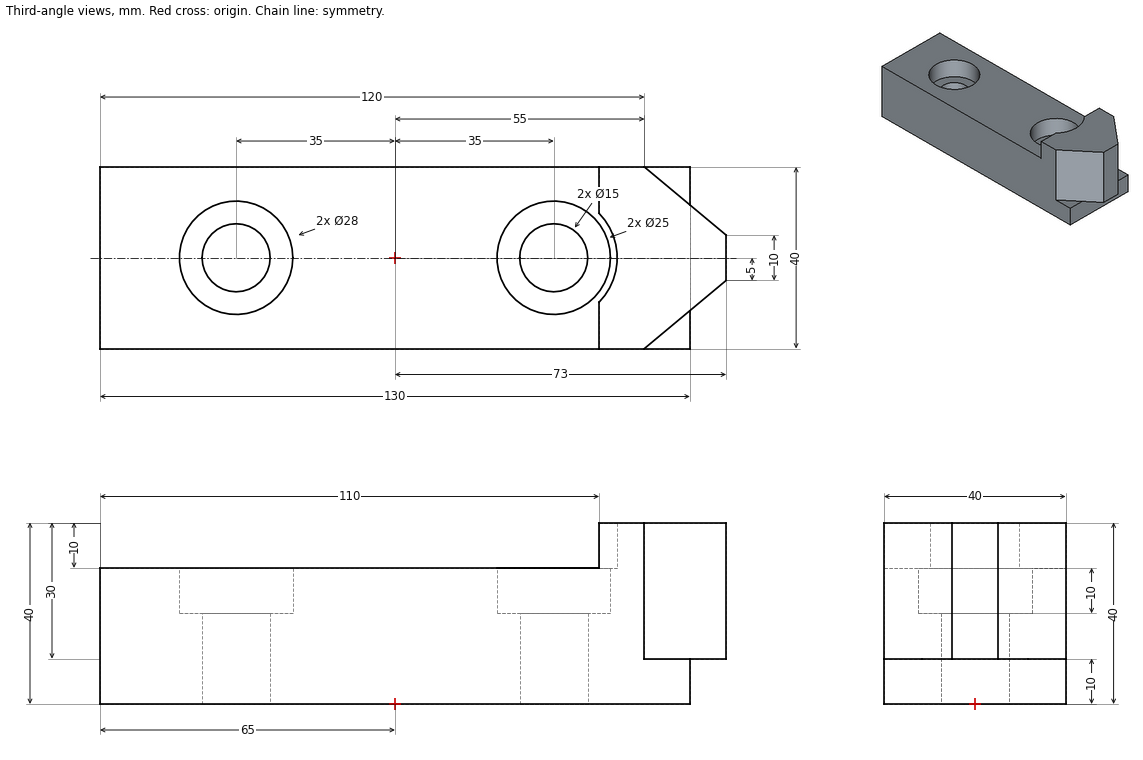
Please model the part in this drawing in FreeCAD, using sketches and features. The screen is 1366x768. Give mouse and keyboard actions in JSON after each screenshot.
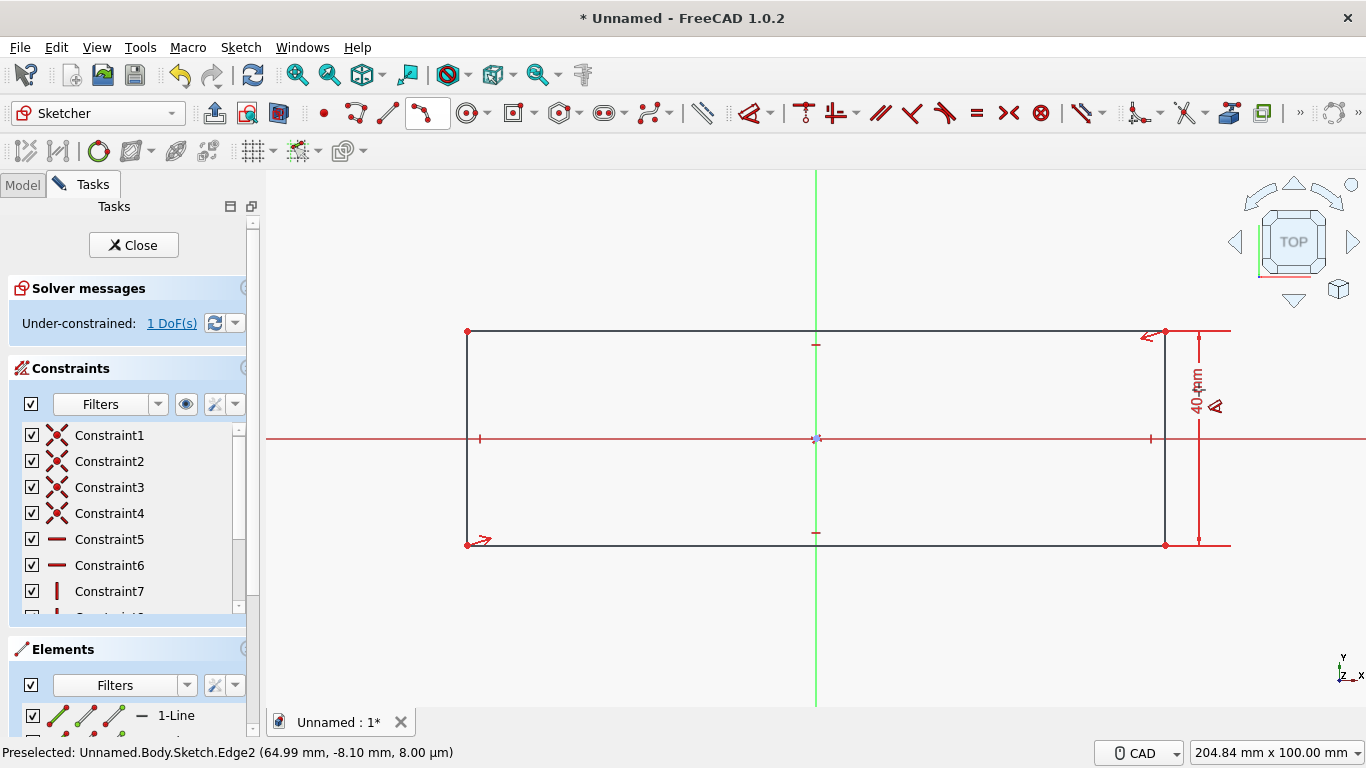
{"action": "left_click", "coordinate": [676, 546]}
{"action": "left_click", "coordinate": [655, 580]}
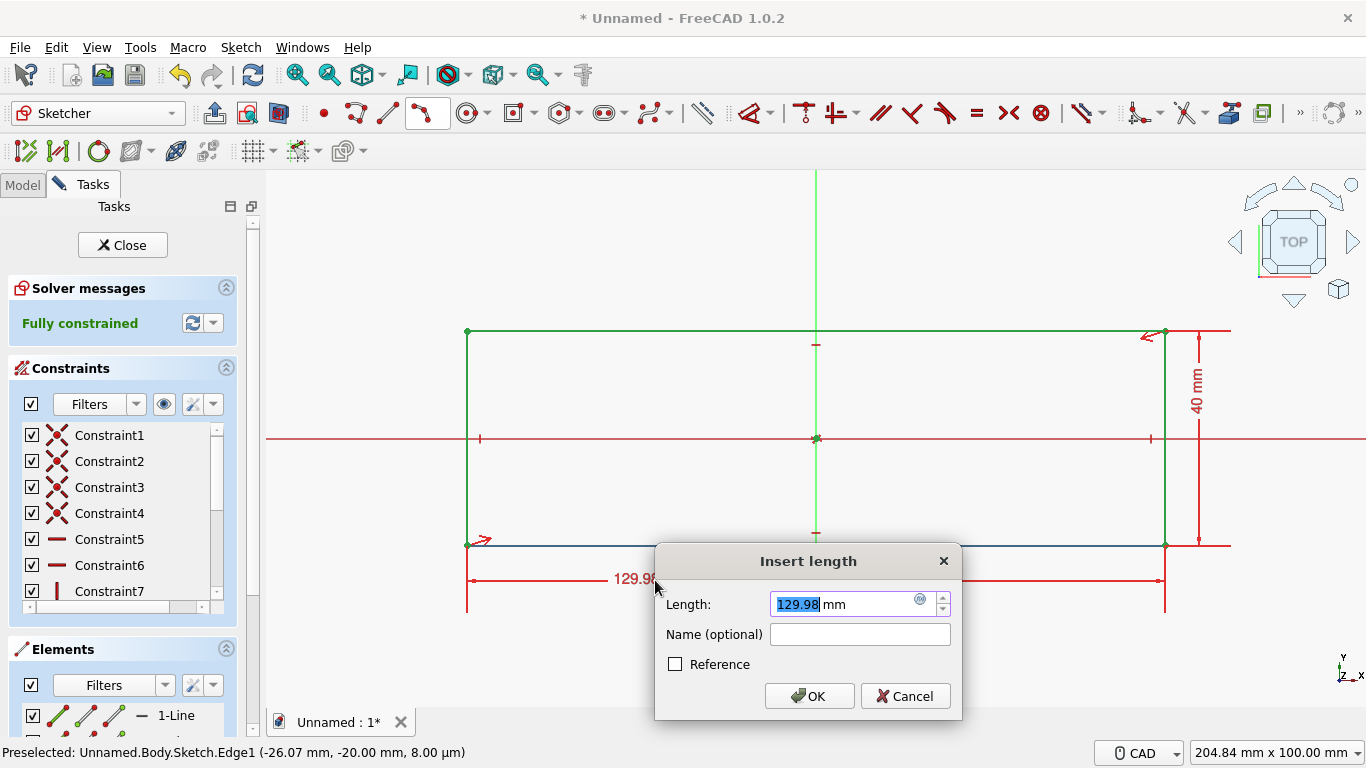
{"action": "type", "text": "130"}
{"action": "key", "text": "Return"}
{"action": "key", "text": "Escape"}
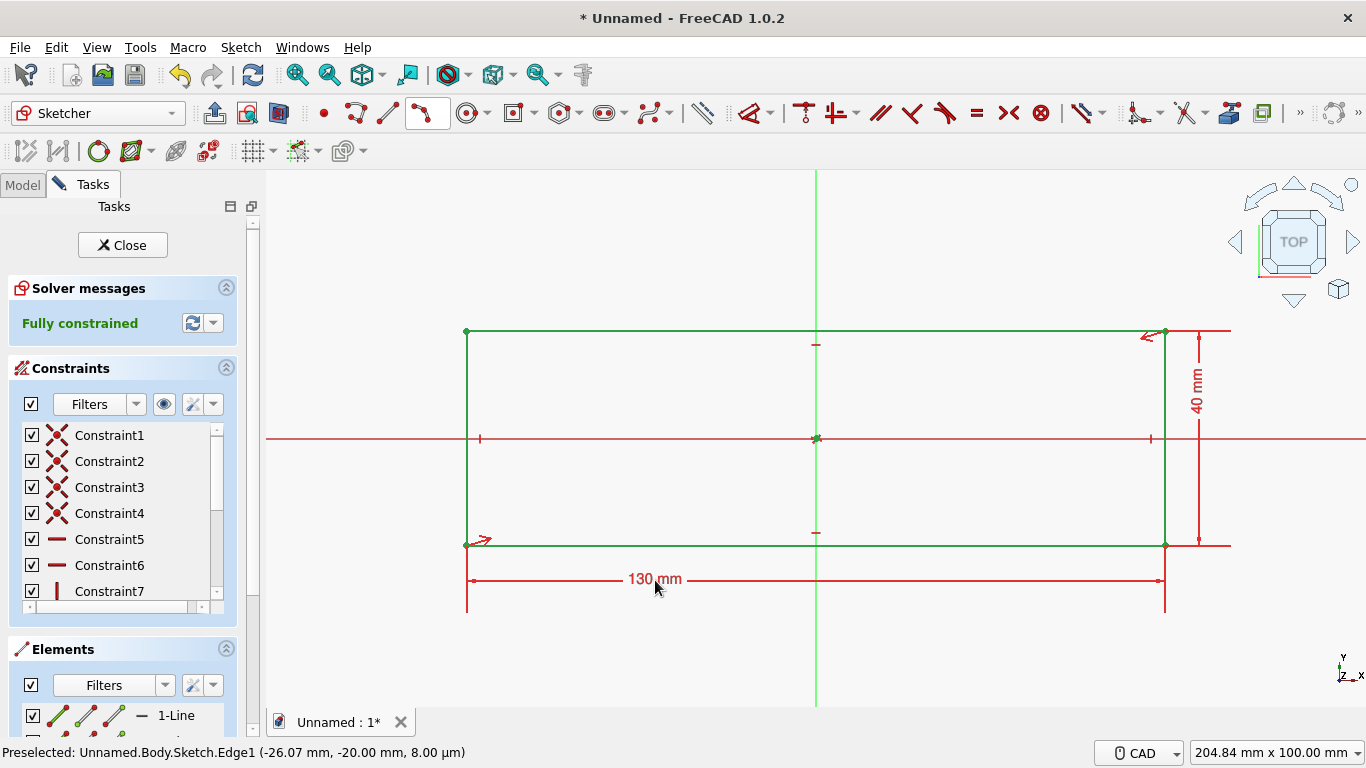
{"action": "left_click", "coordinate": [123, 245]}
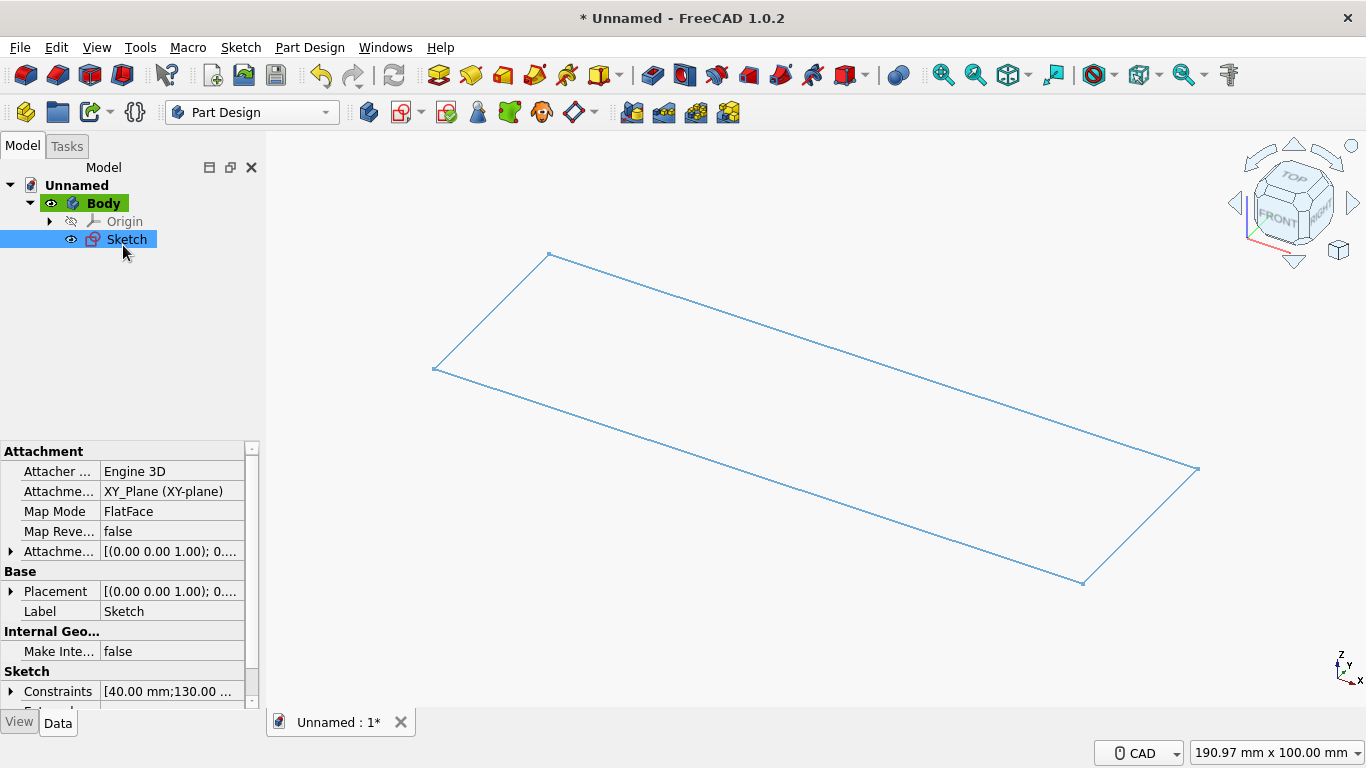
{"action": "left_click", "coordinate": [440, 76]}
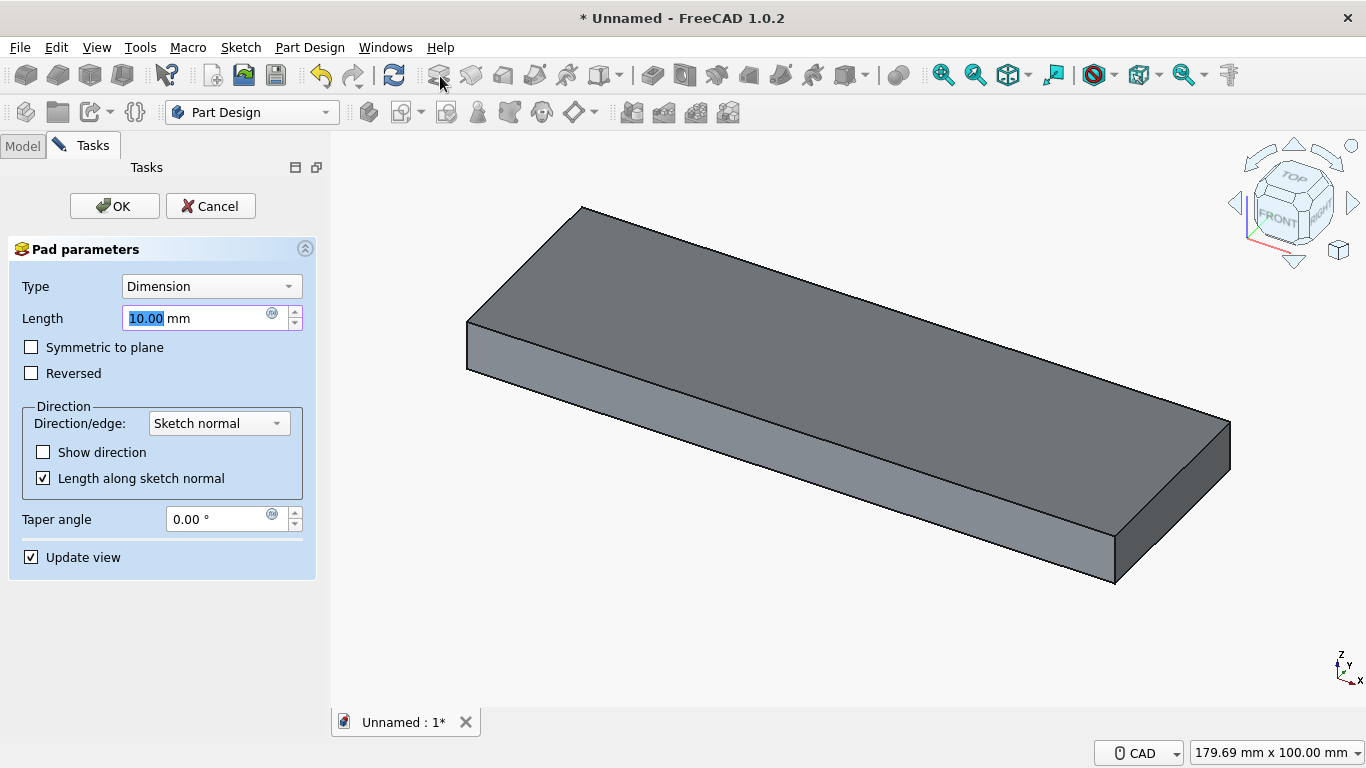
{"action": "type", "text": "10"}
{"action": "key", "text": "Tab"}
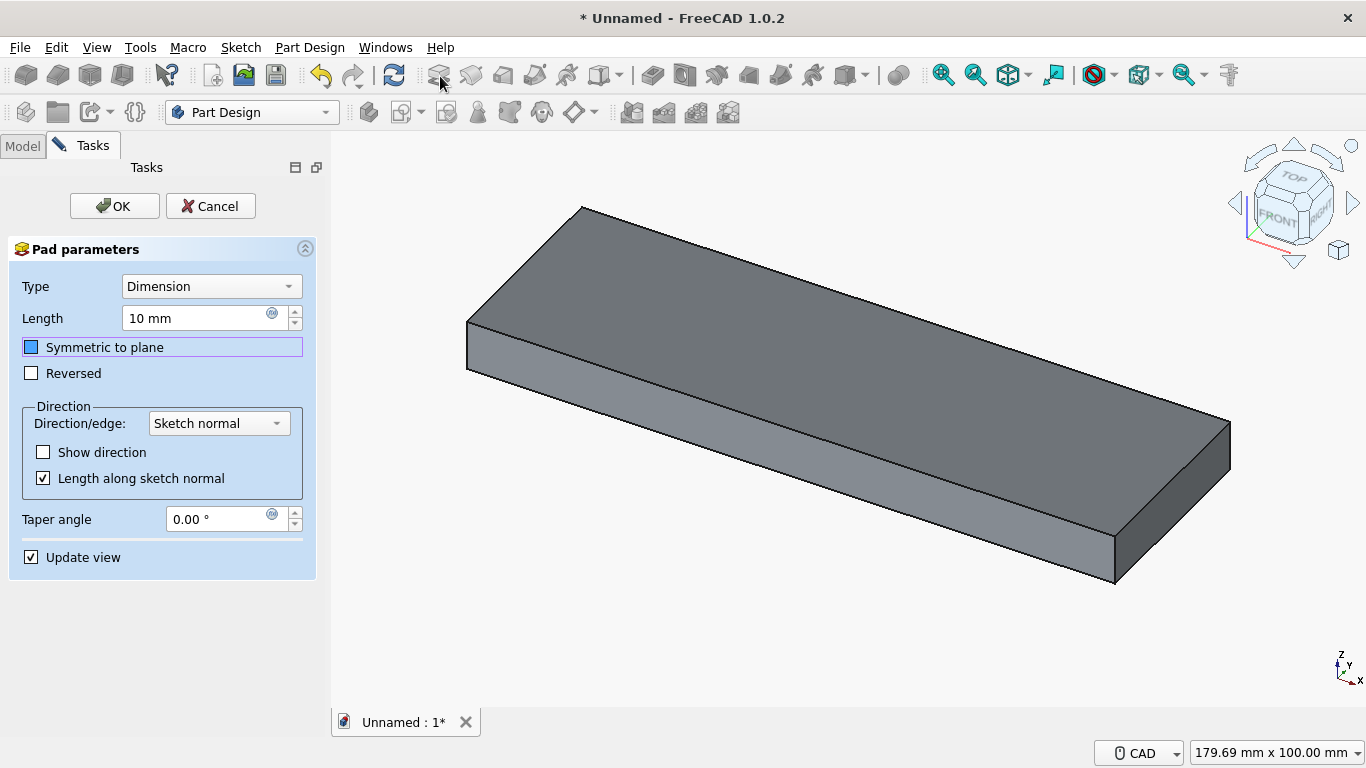
{"action": "left_click", "coordinate": [115, 206]}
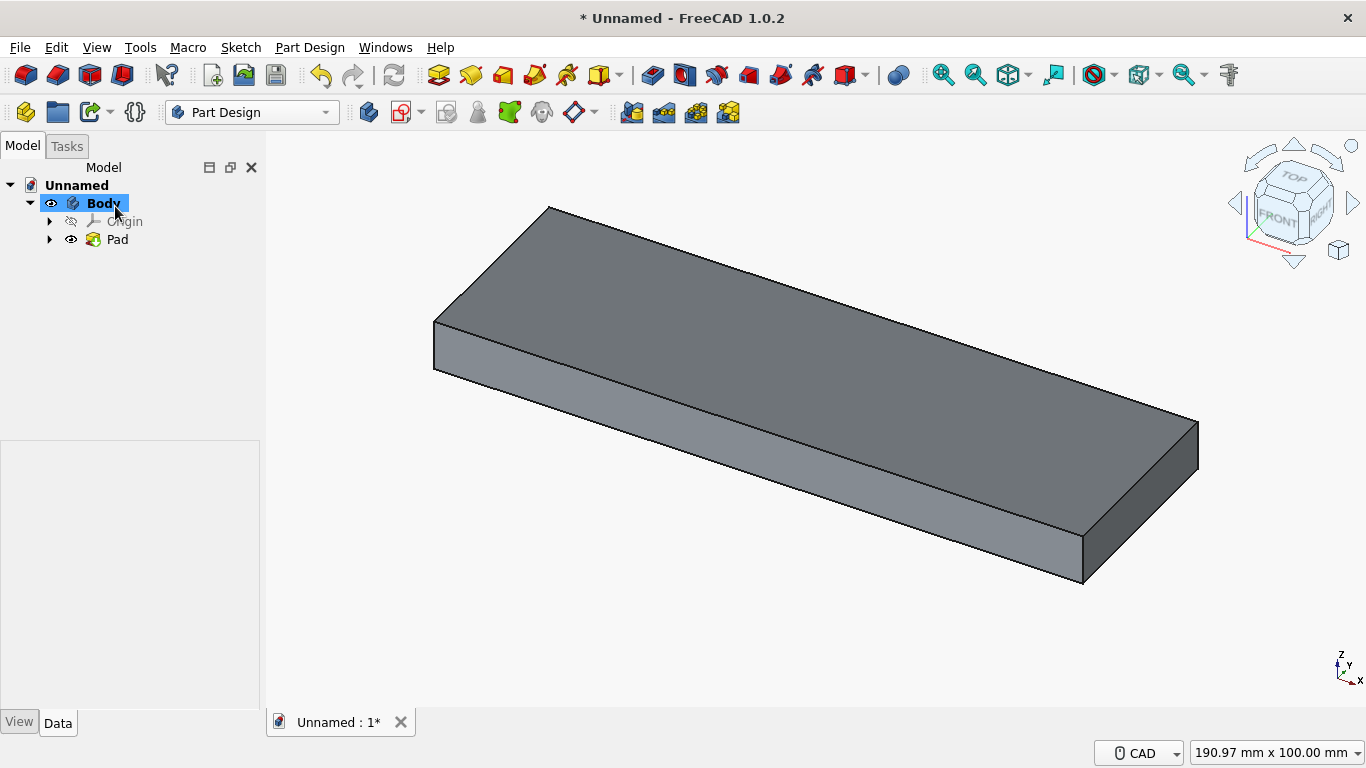
{"action": "left_click", "coordinate": [1001, 432]}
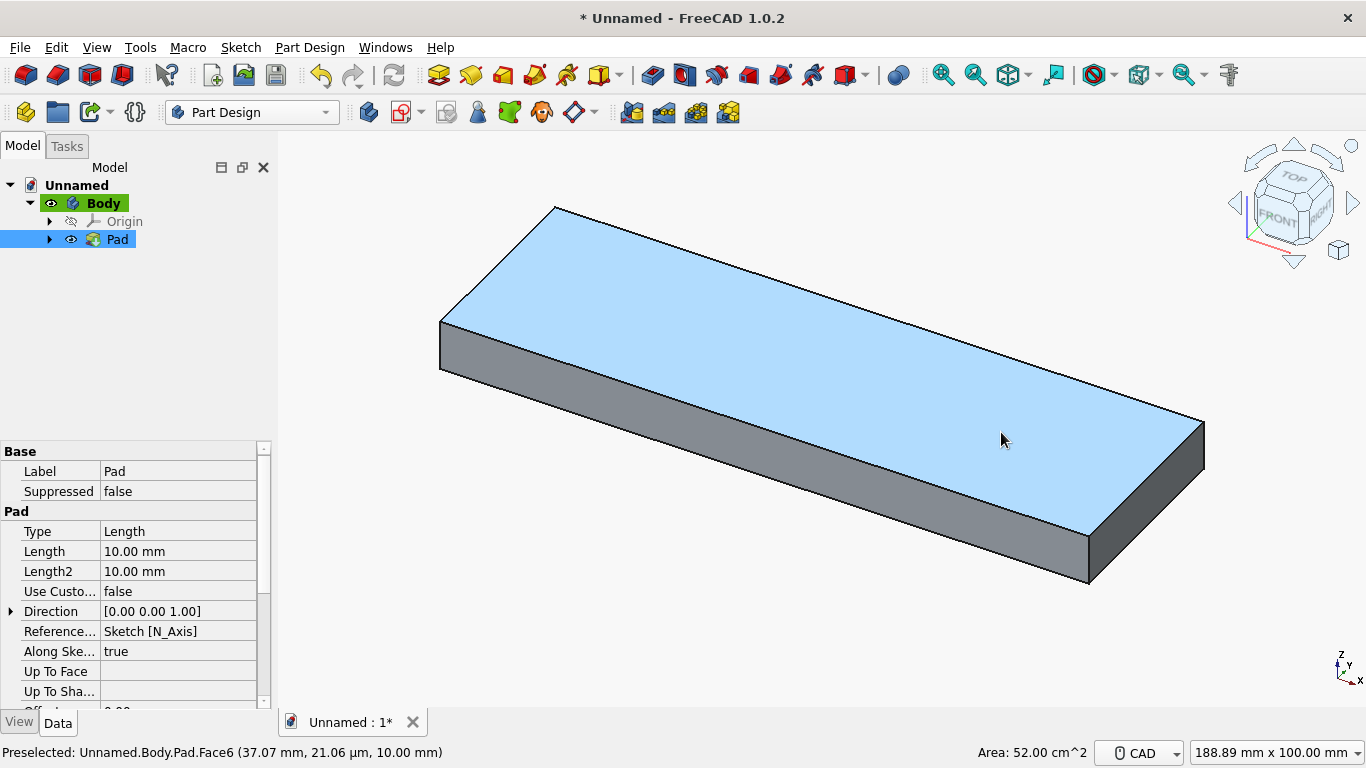
{"action": "left_click", "coordinate": [402, 112]}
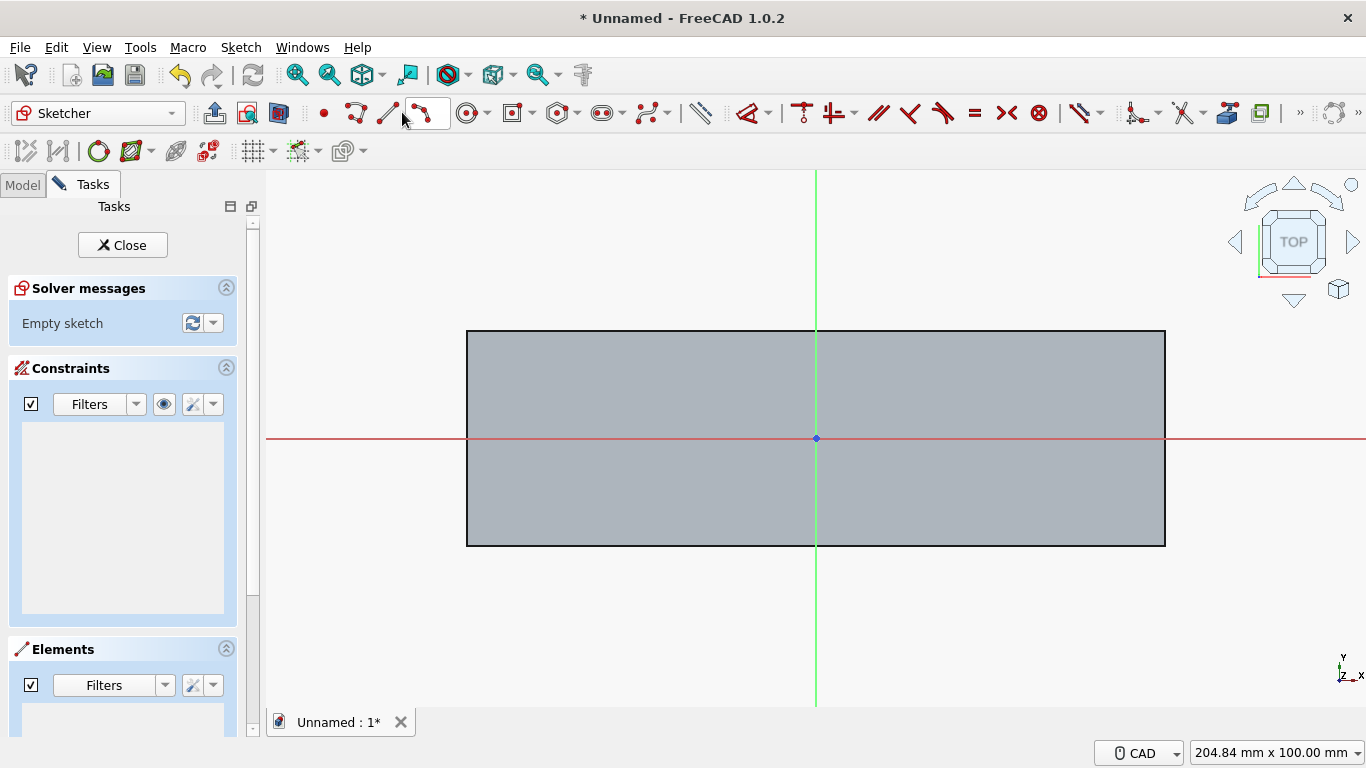
{"action": "scroll", "coordinate": [341, 439], "scroll_direction": "down", "scroll_amount": 1}